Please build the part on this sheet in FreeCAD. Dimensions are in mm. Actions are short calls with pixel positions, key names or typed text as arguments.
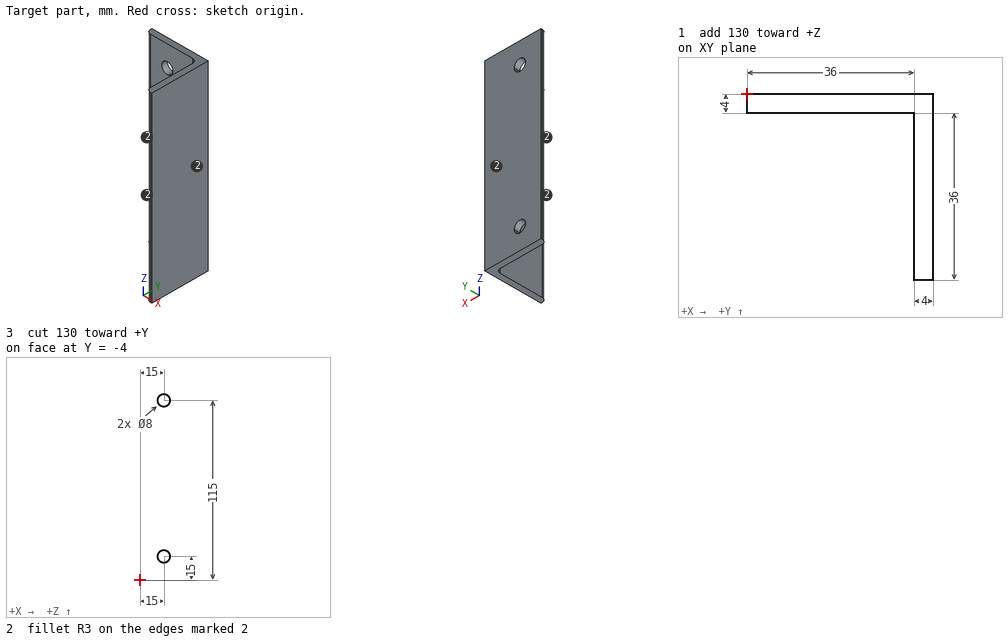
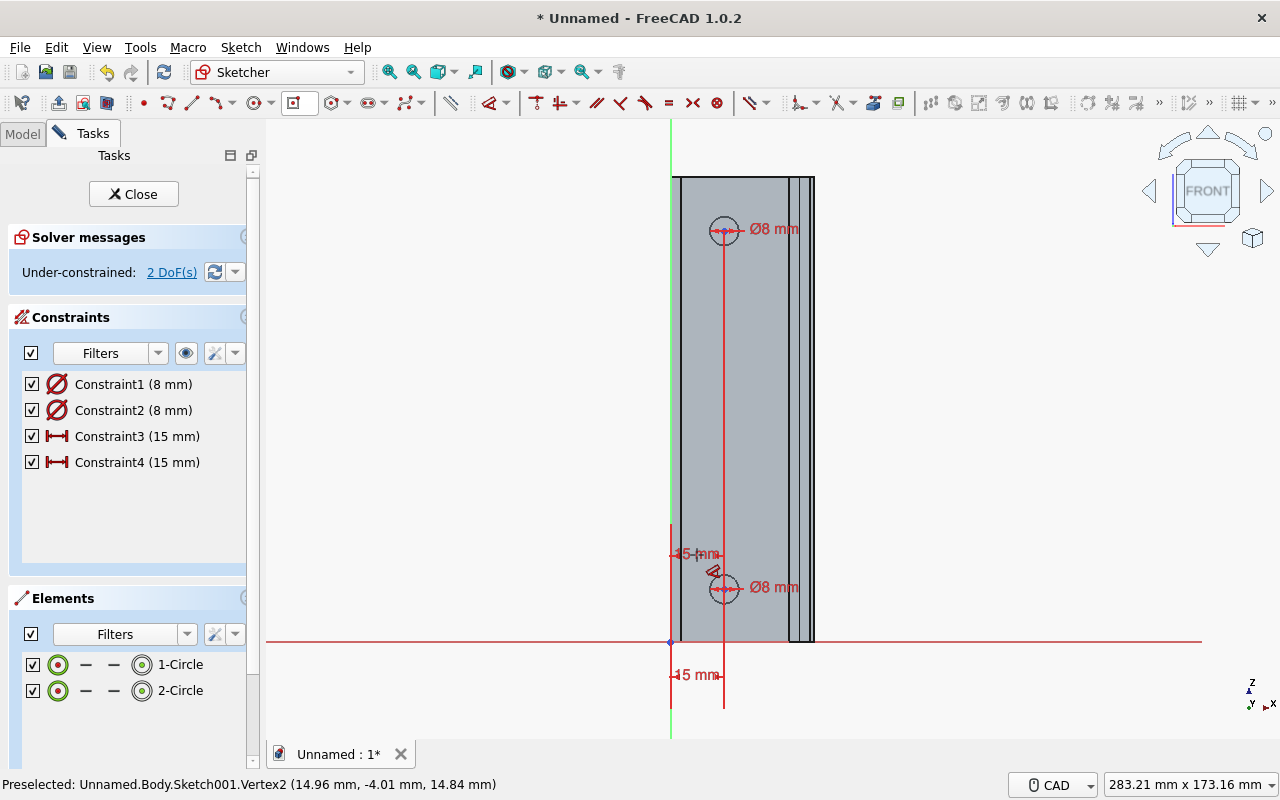
click(724, 589)
click(637, 616)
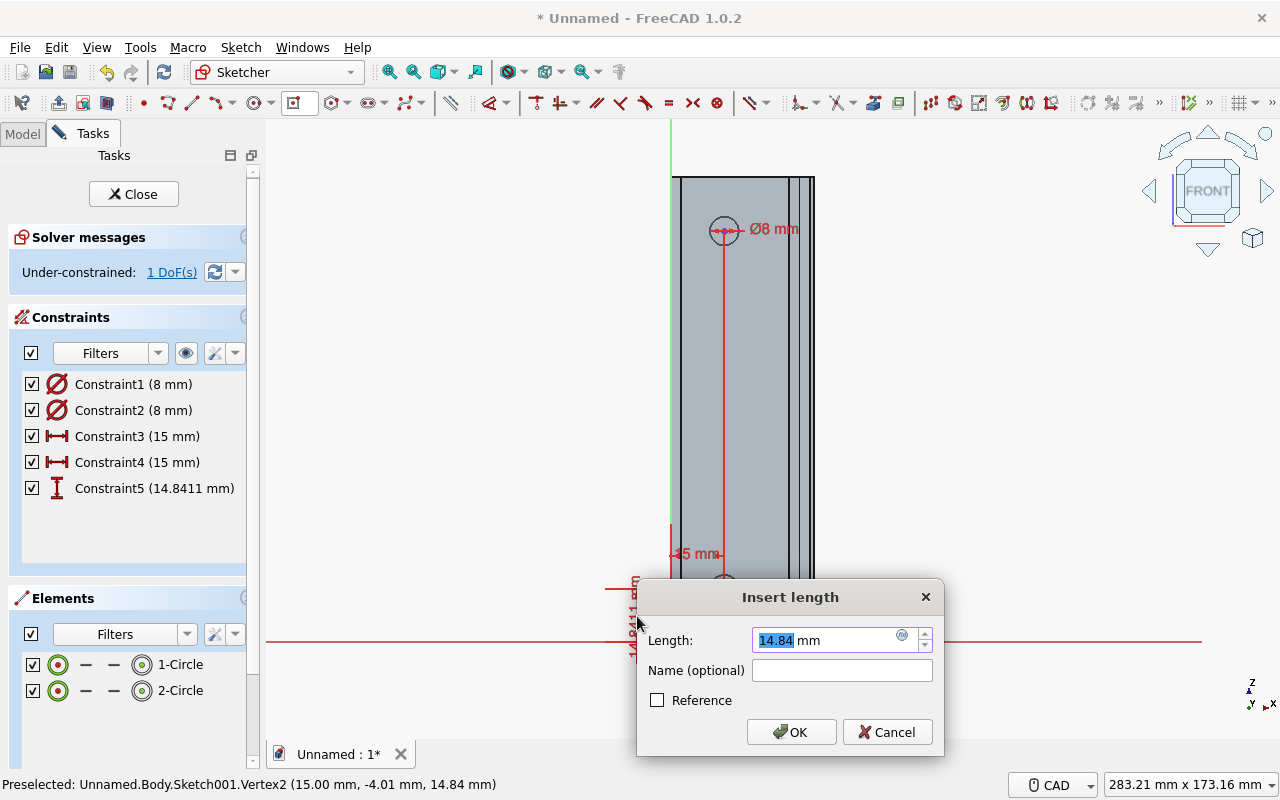
text(15)
key(Return)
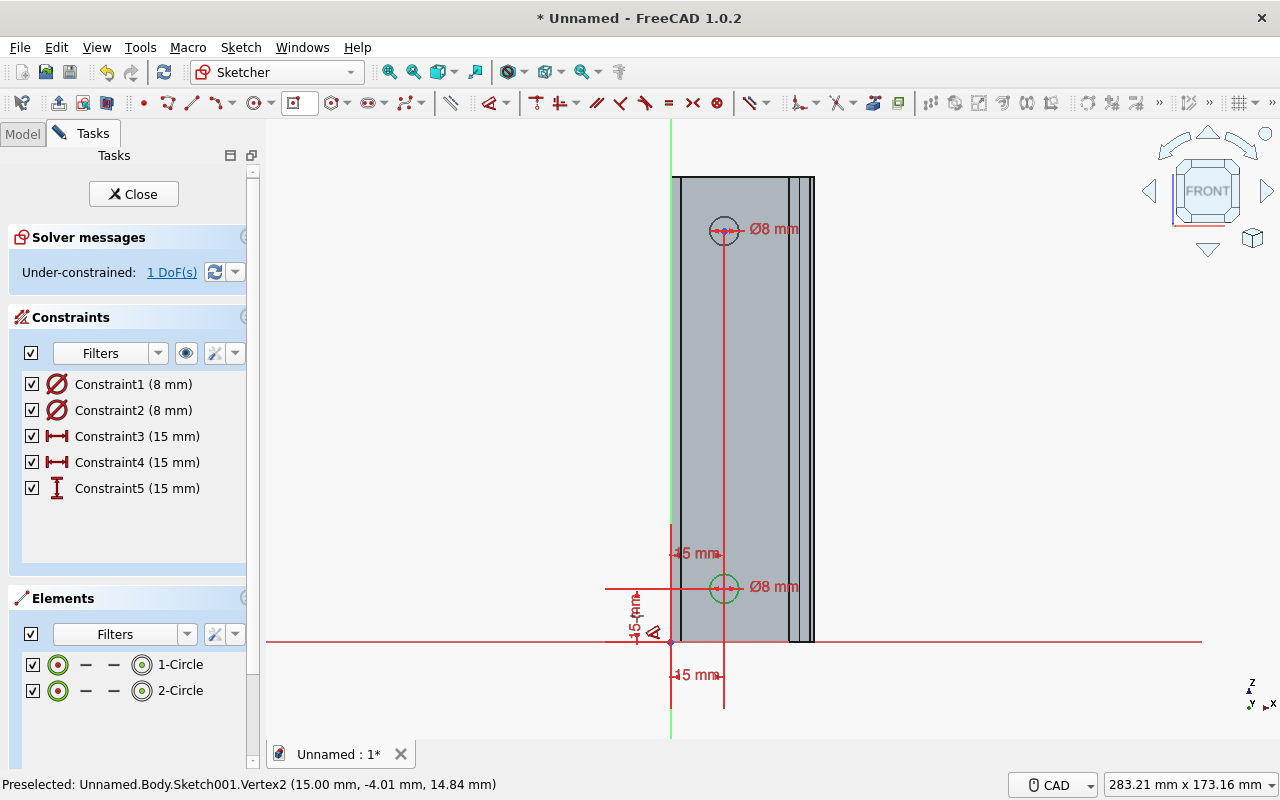
click(724, 231)
click(637, 437)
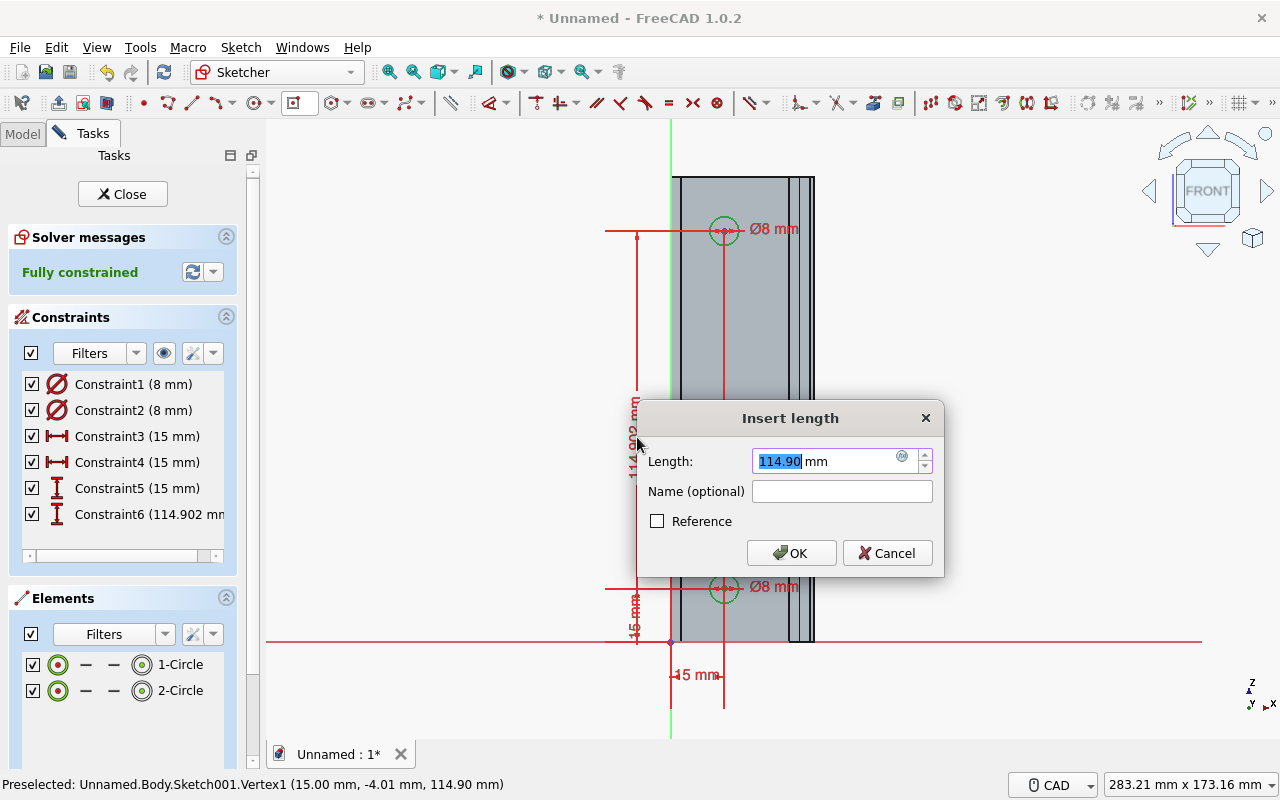
text(115)
key(Return)
key(Escape)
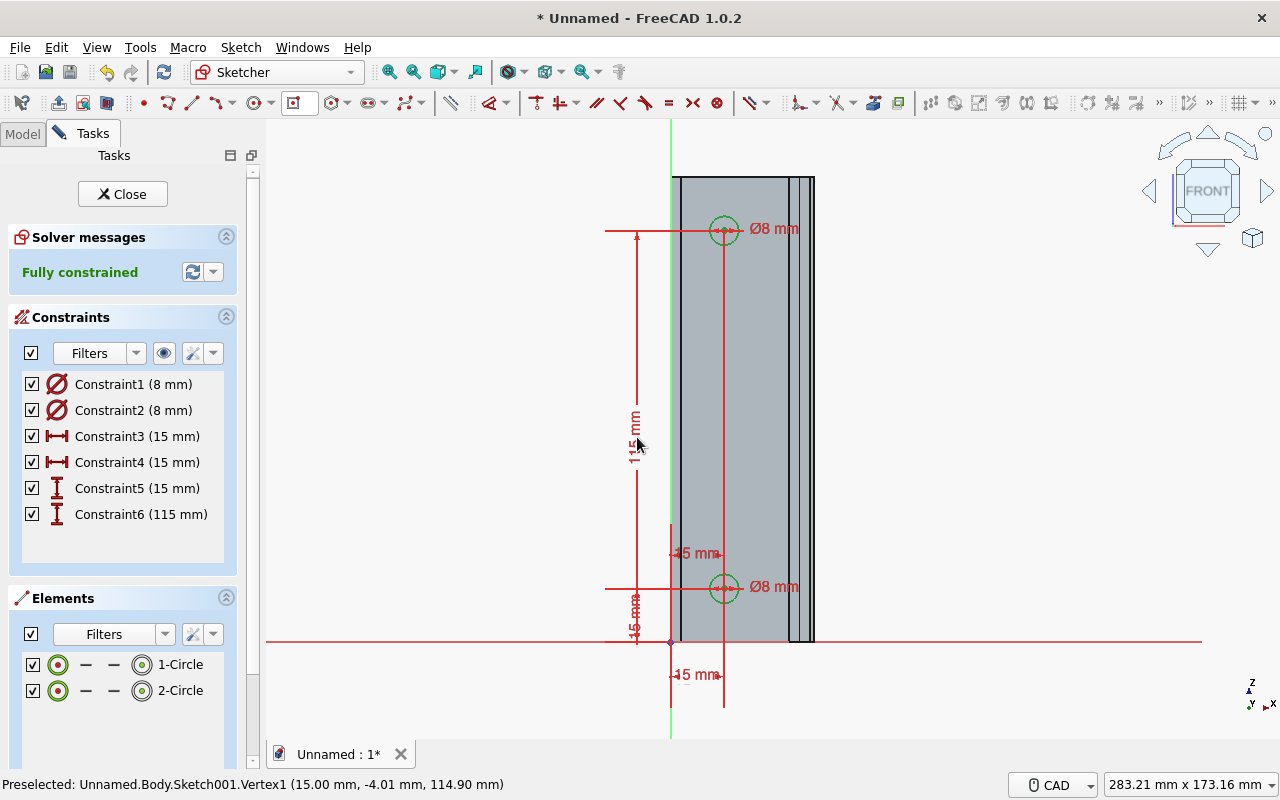
click(123, 194)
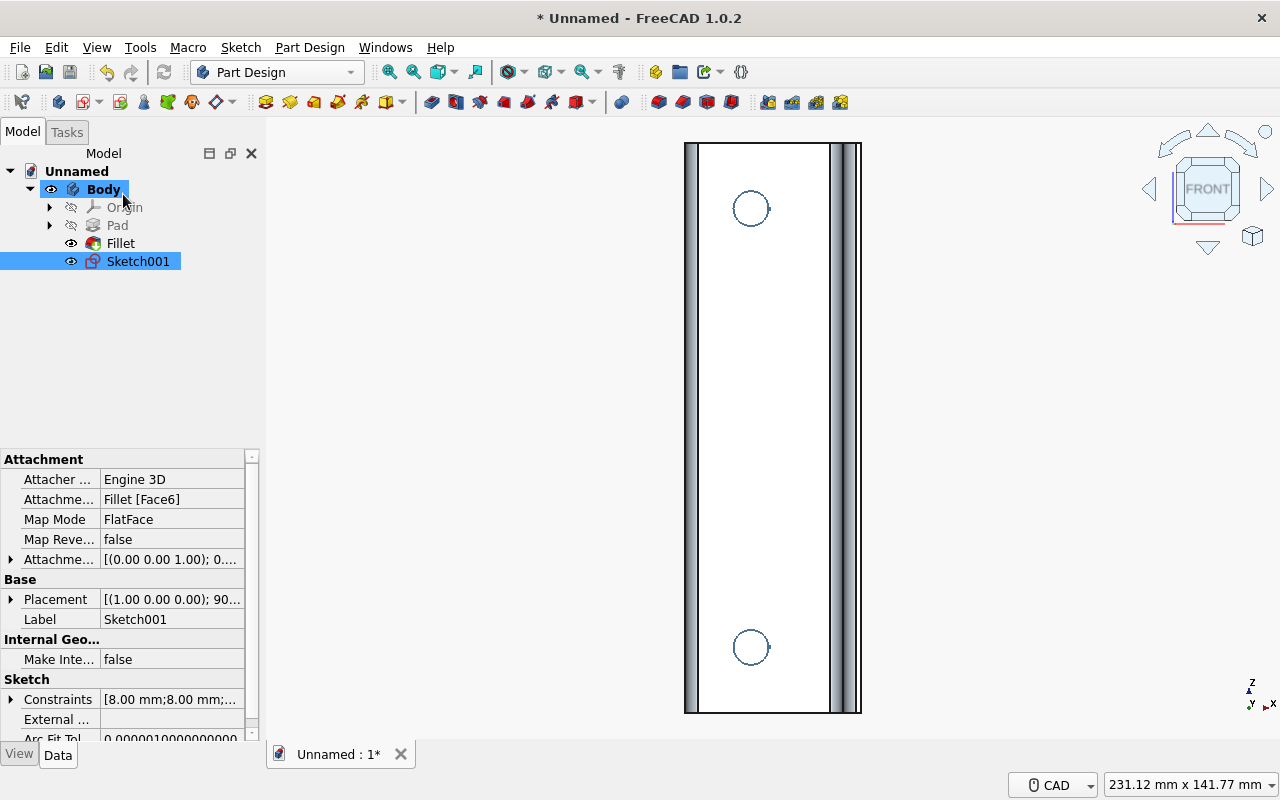
click(432, 102)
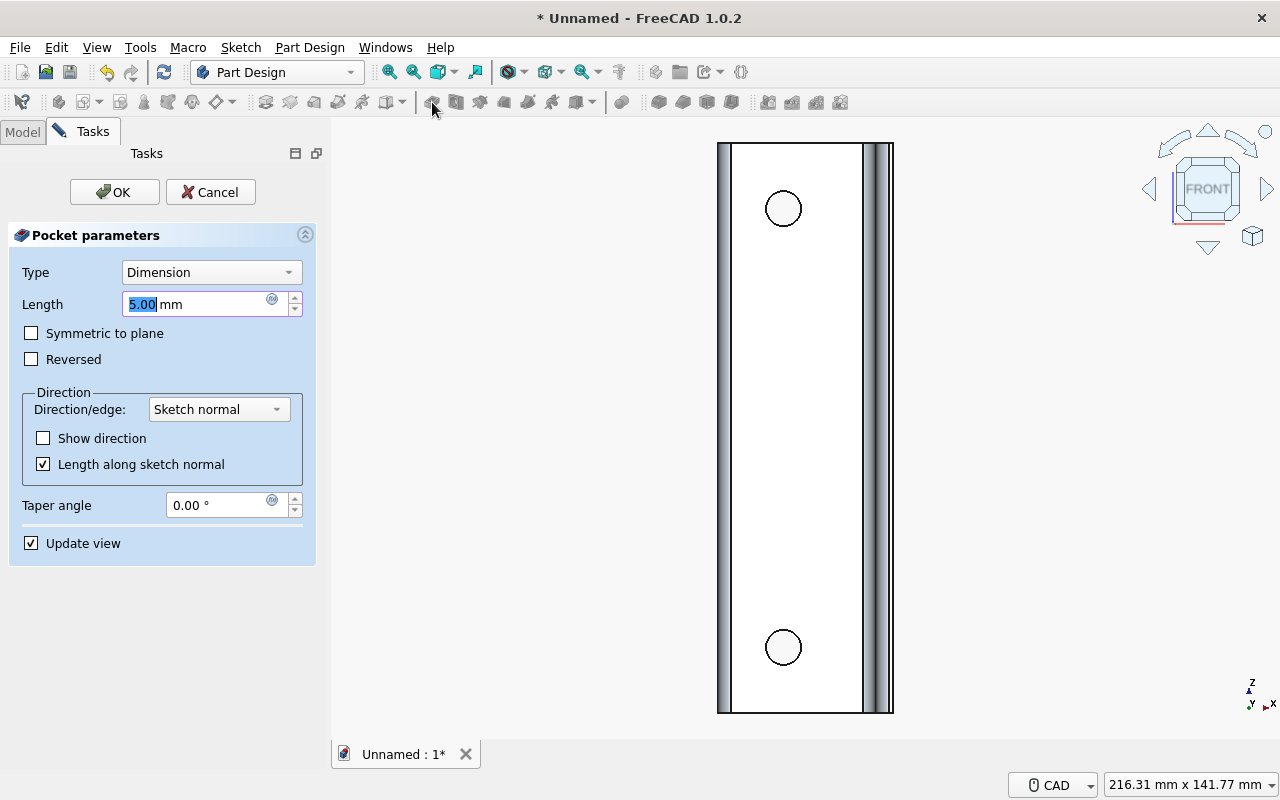
text(130)
key(Tab)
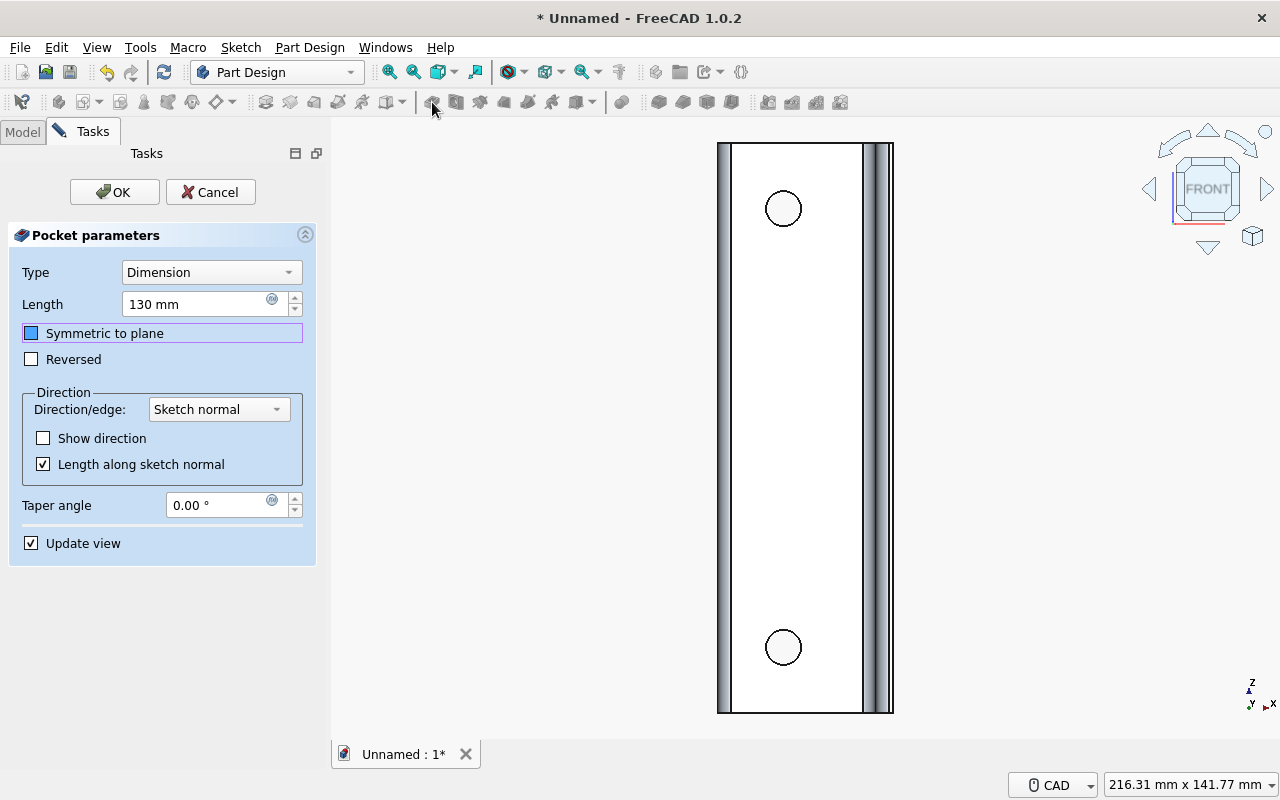
click(115, 192)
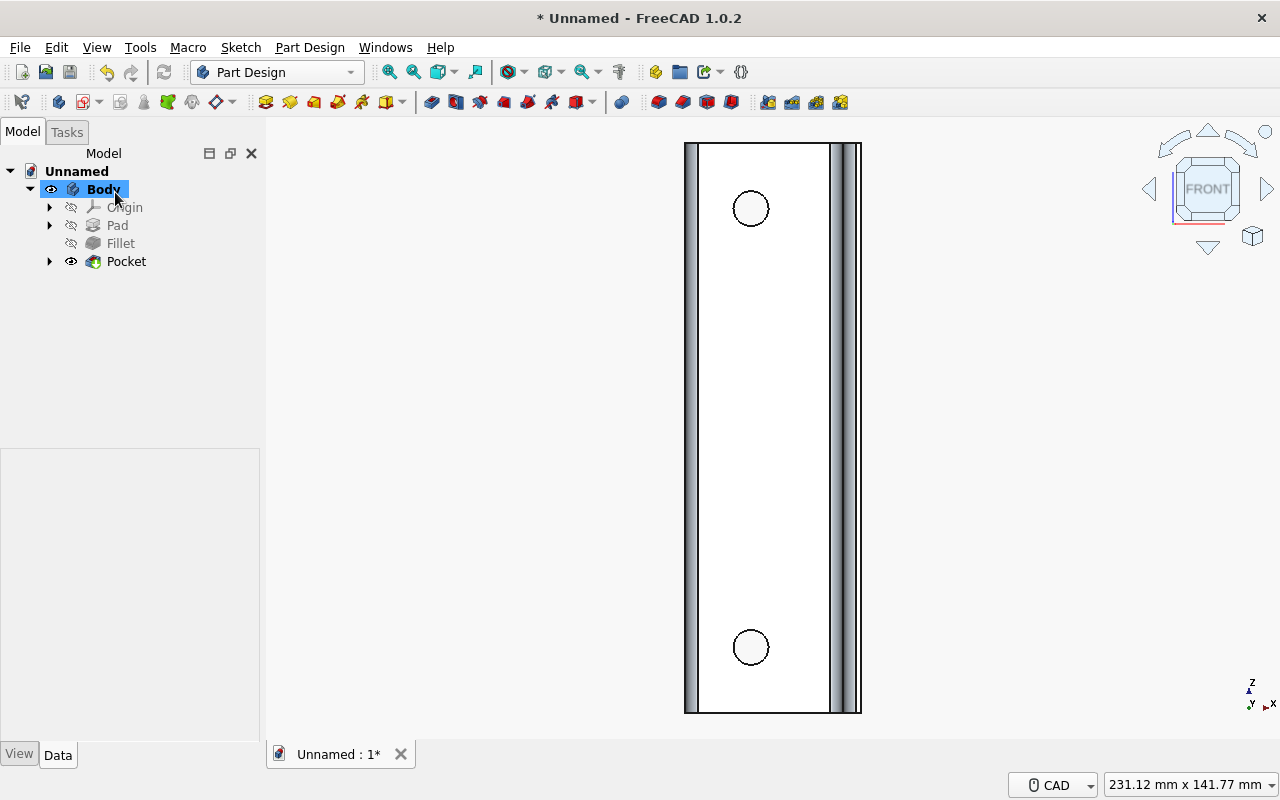
key(0)